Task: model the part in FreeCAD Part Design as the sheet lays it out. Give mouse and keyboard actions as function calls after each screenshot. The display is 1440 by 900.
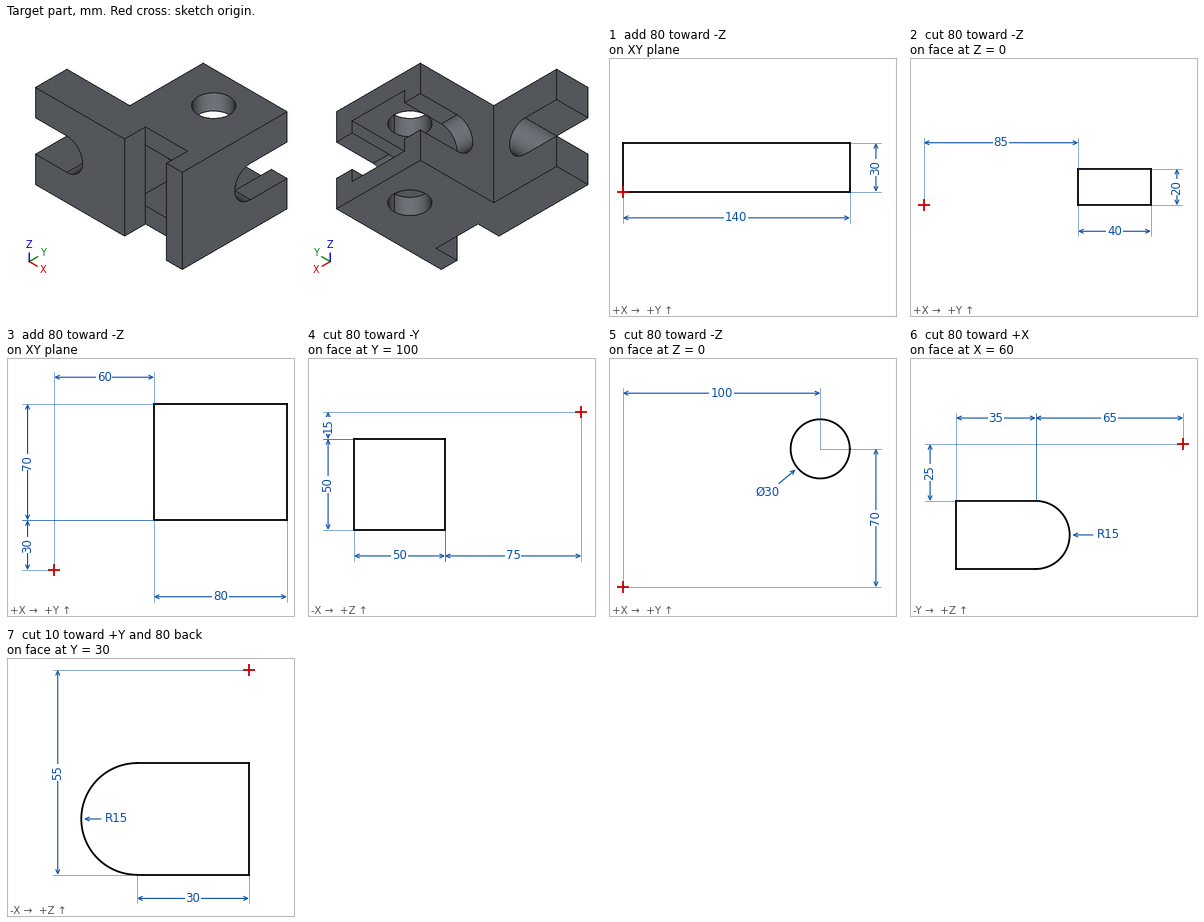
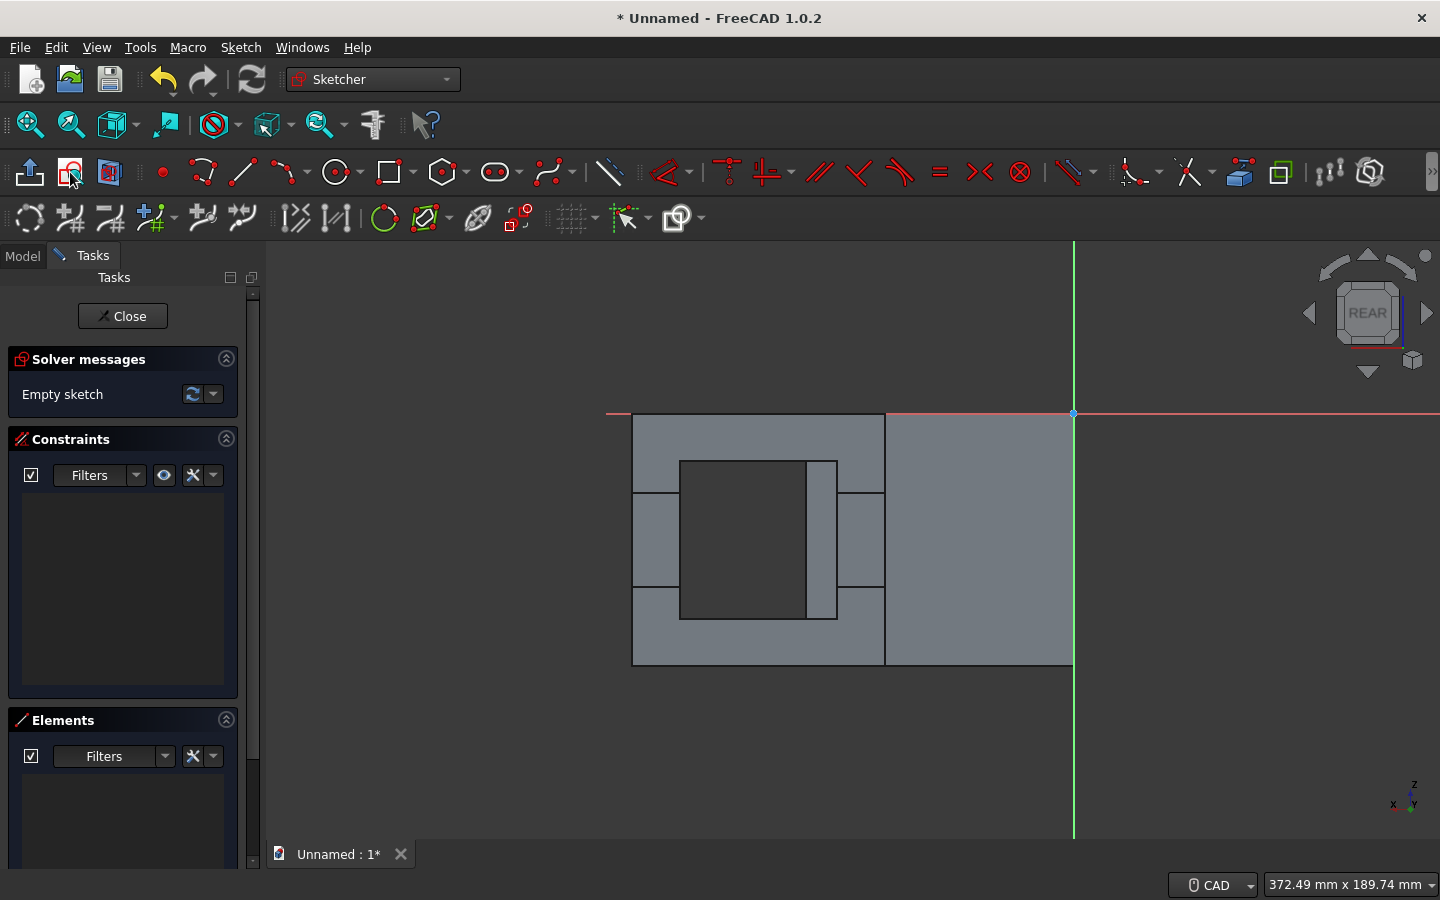
scroll(1181, 468, up, 4)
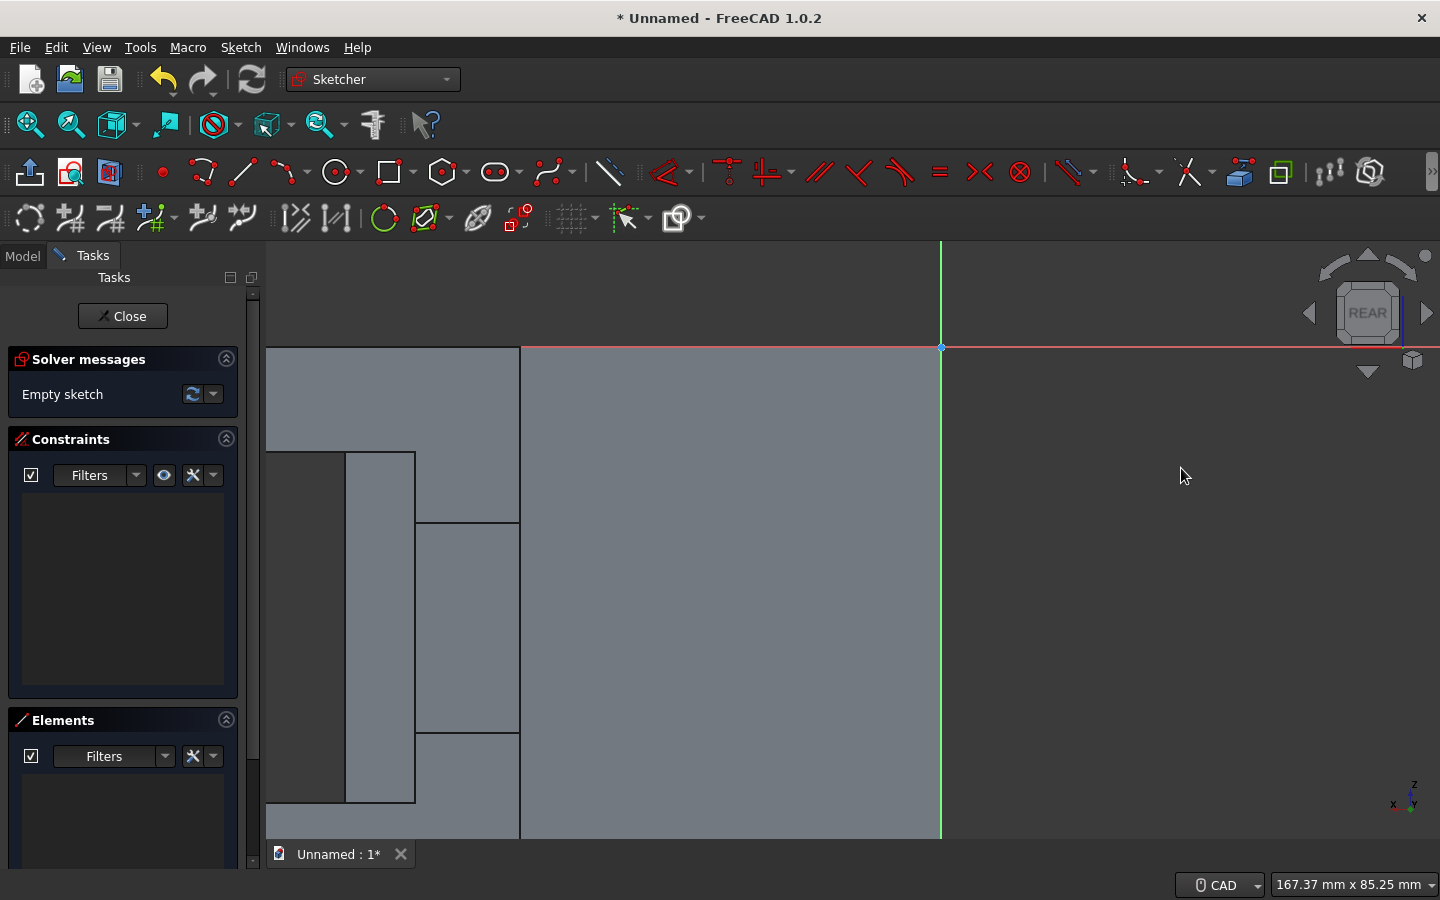
key(g)
key(m)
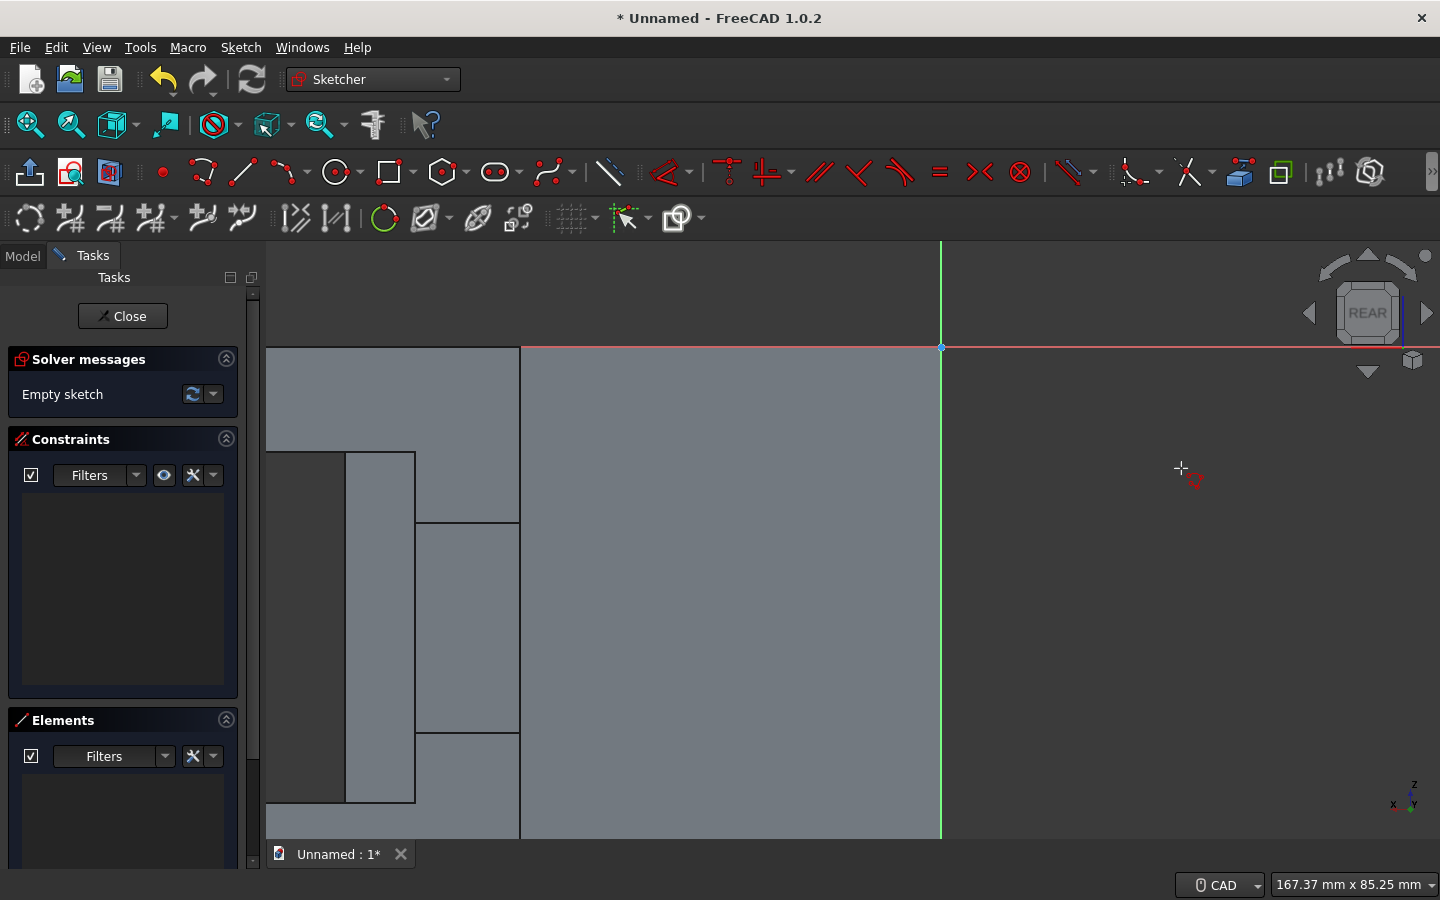
click(731, 733)
click(941, 733)
click(932, 523)
click(731, 523)
right_click(731, 523)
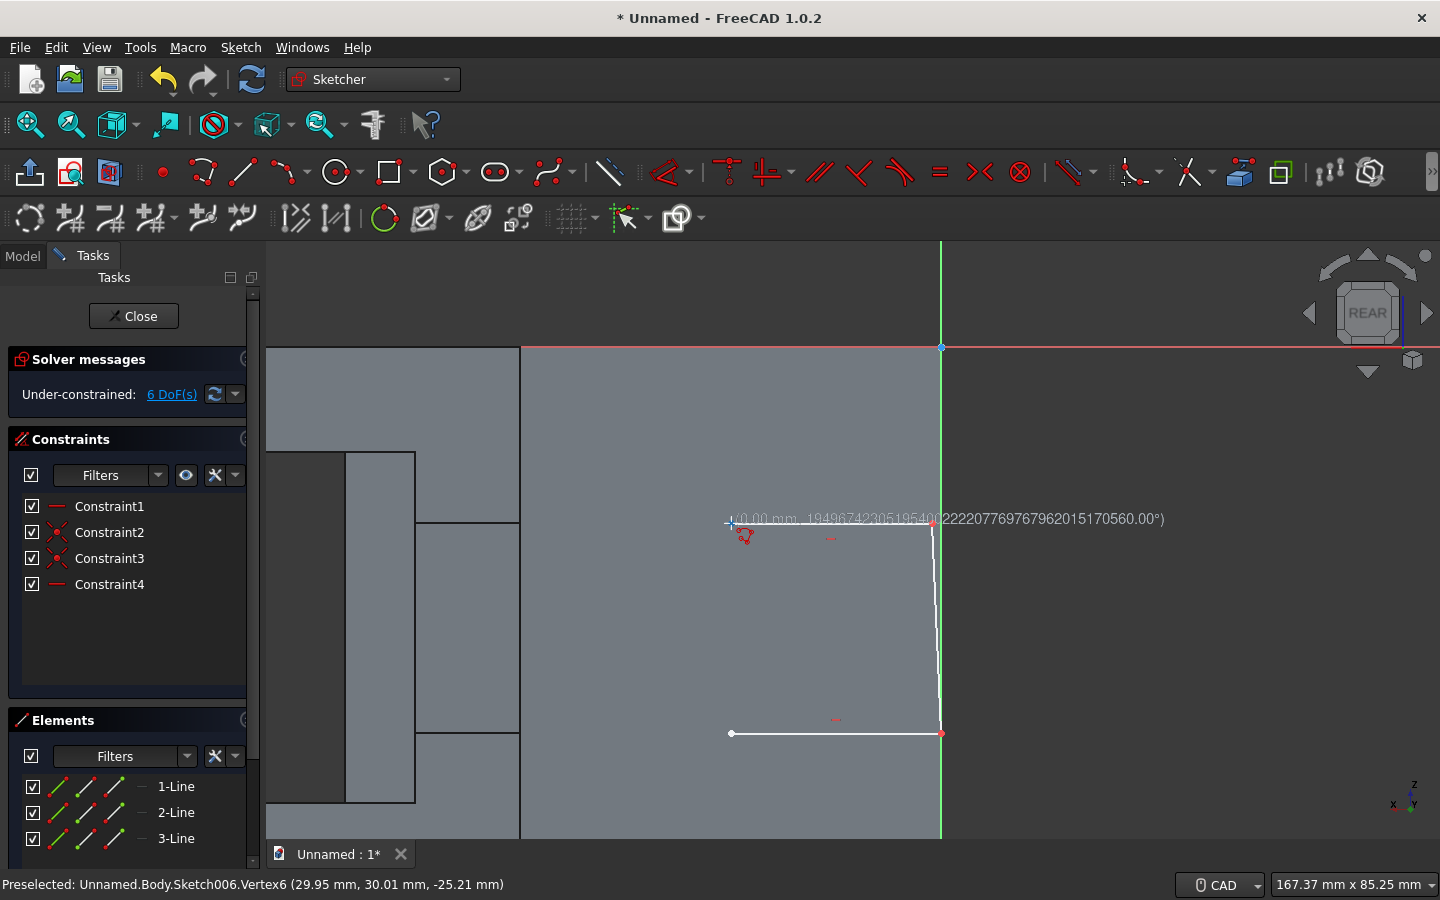
key(g)
key(3)
key(a)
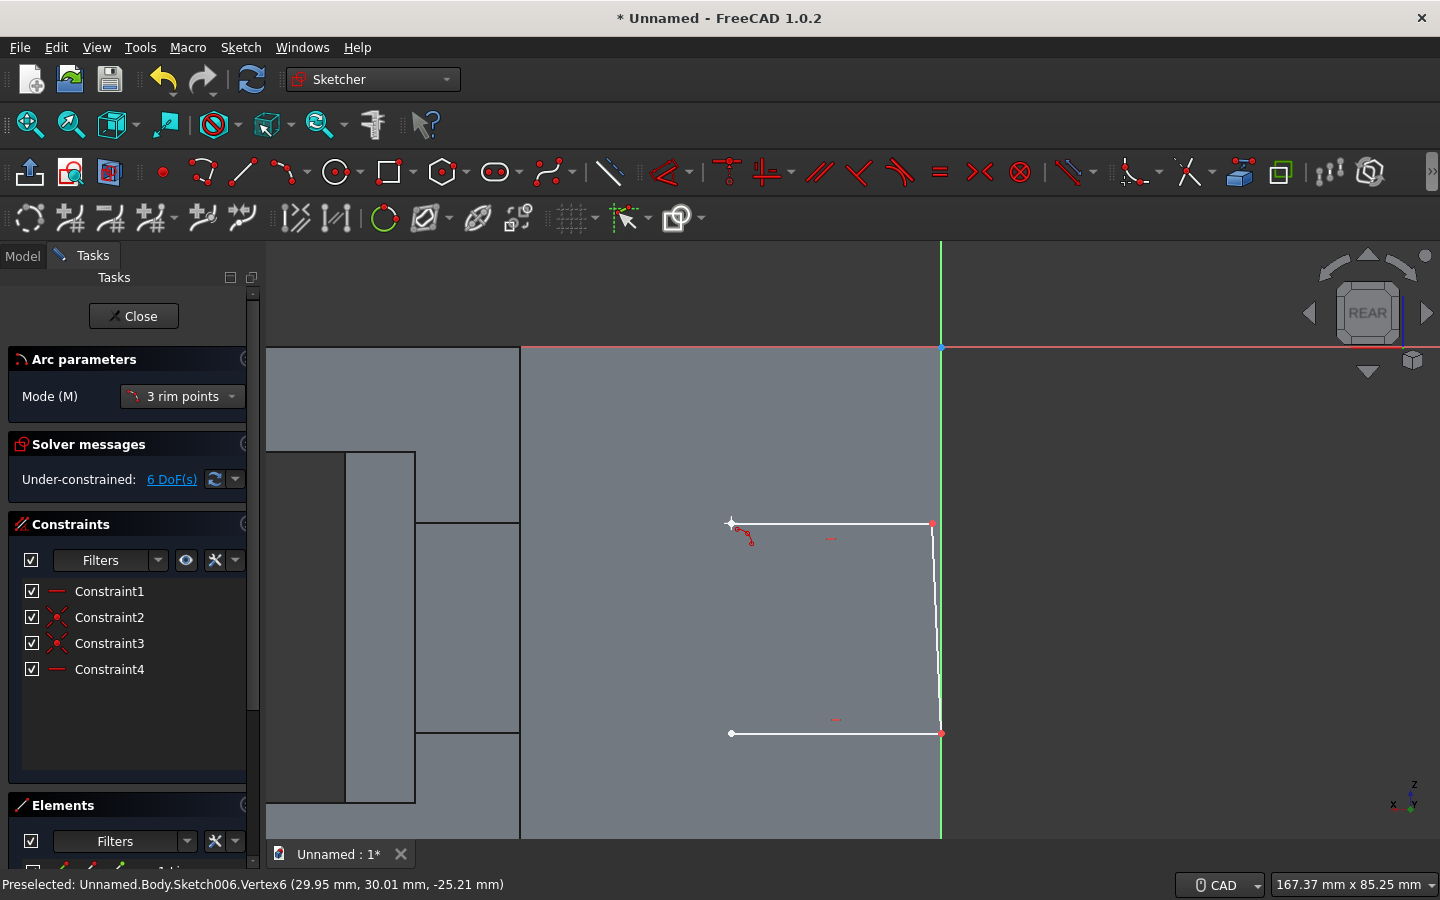
click(731, 524)
click(731, 734)
click(625, 628)
key(Escape)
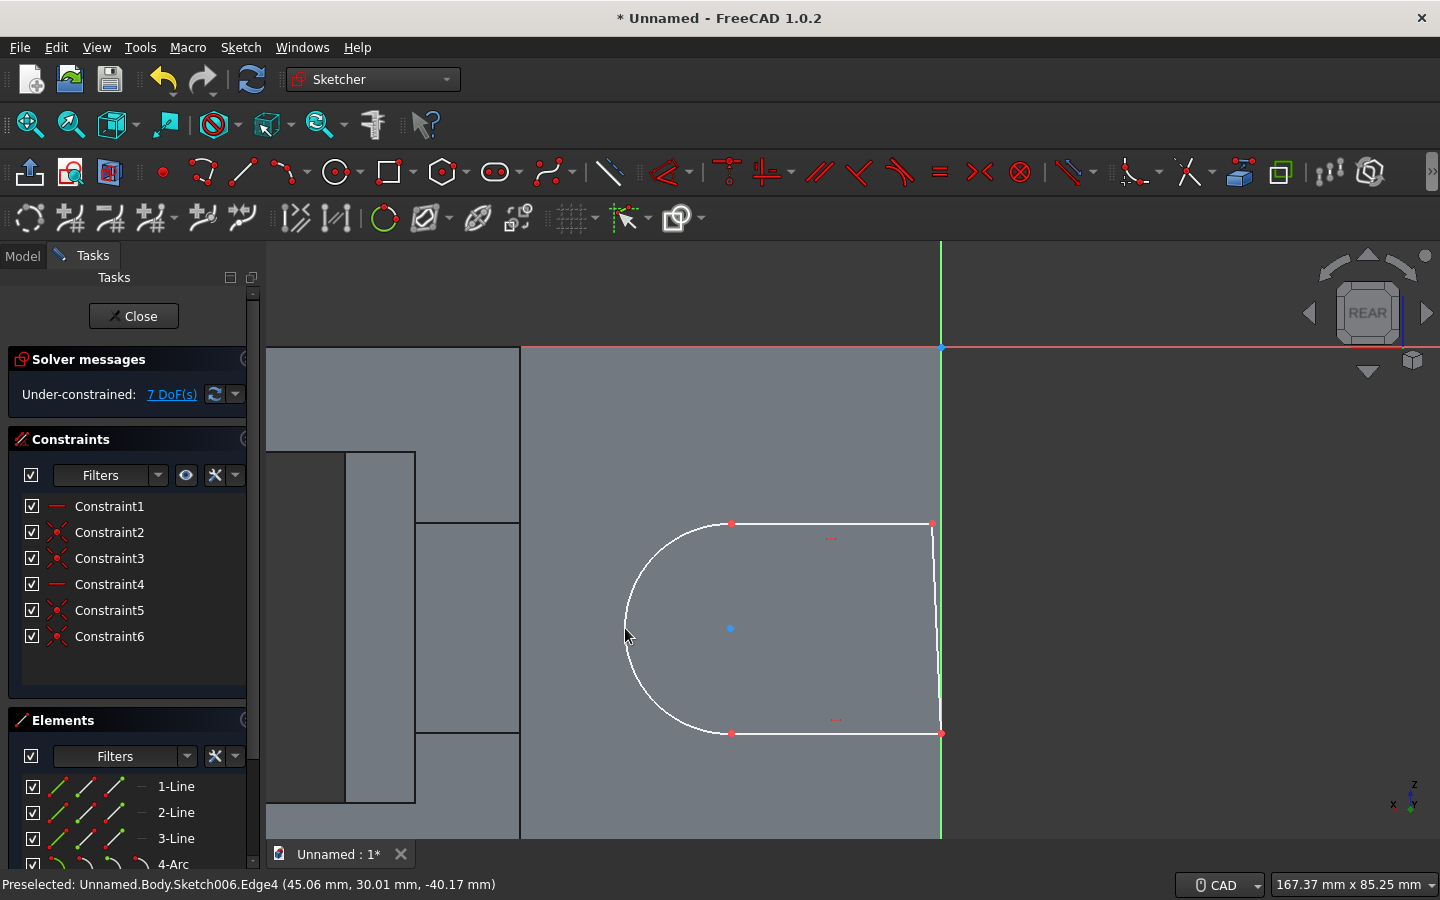
click(794, 734)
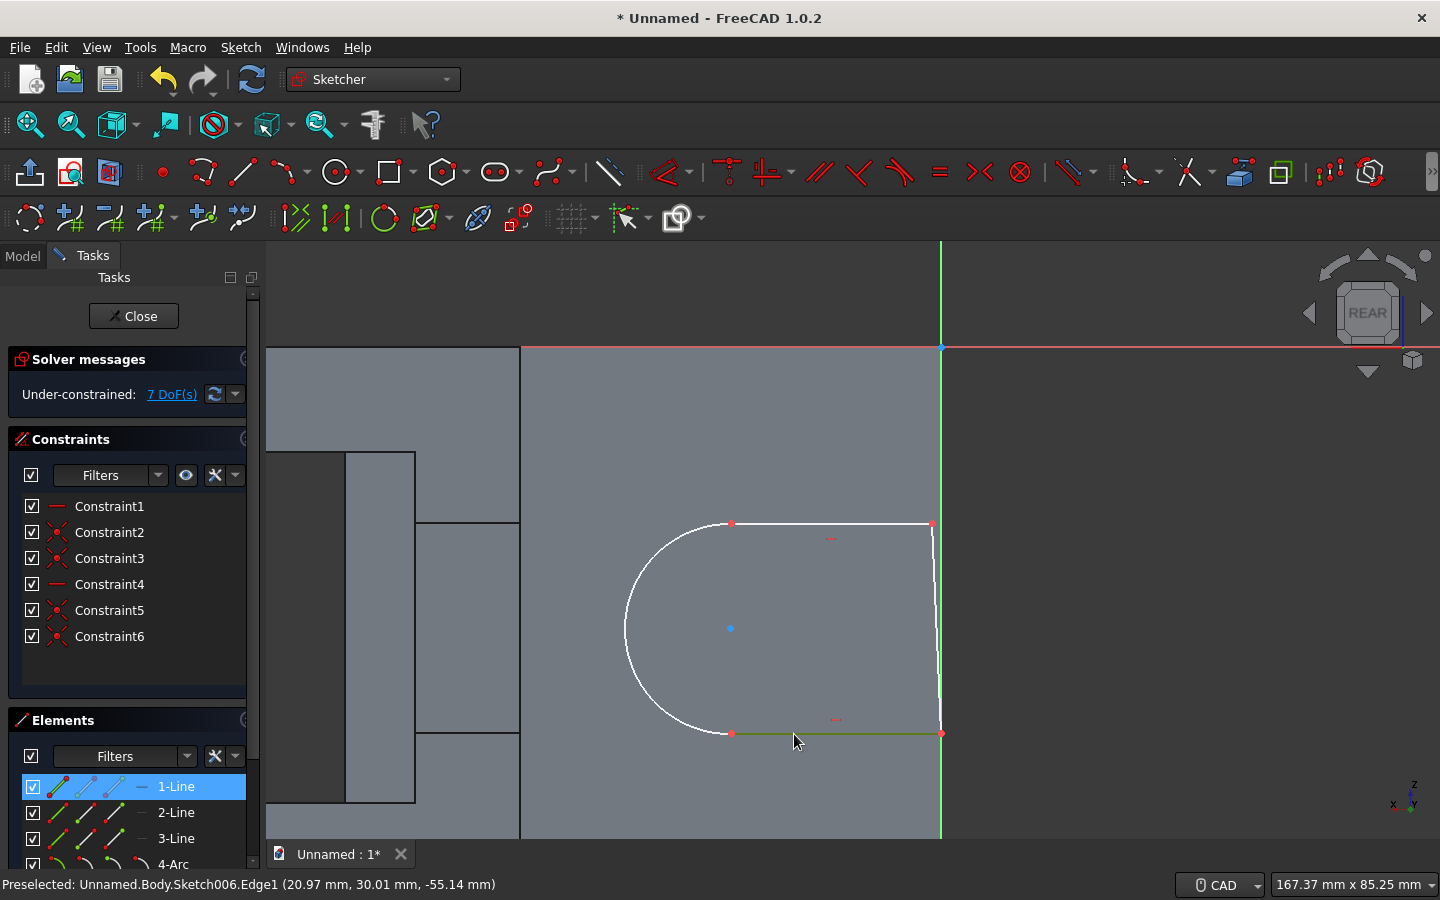
click(645, 567)